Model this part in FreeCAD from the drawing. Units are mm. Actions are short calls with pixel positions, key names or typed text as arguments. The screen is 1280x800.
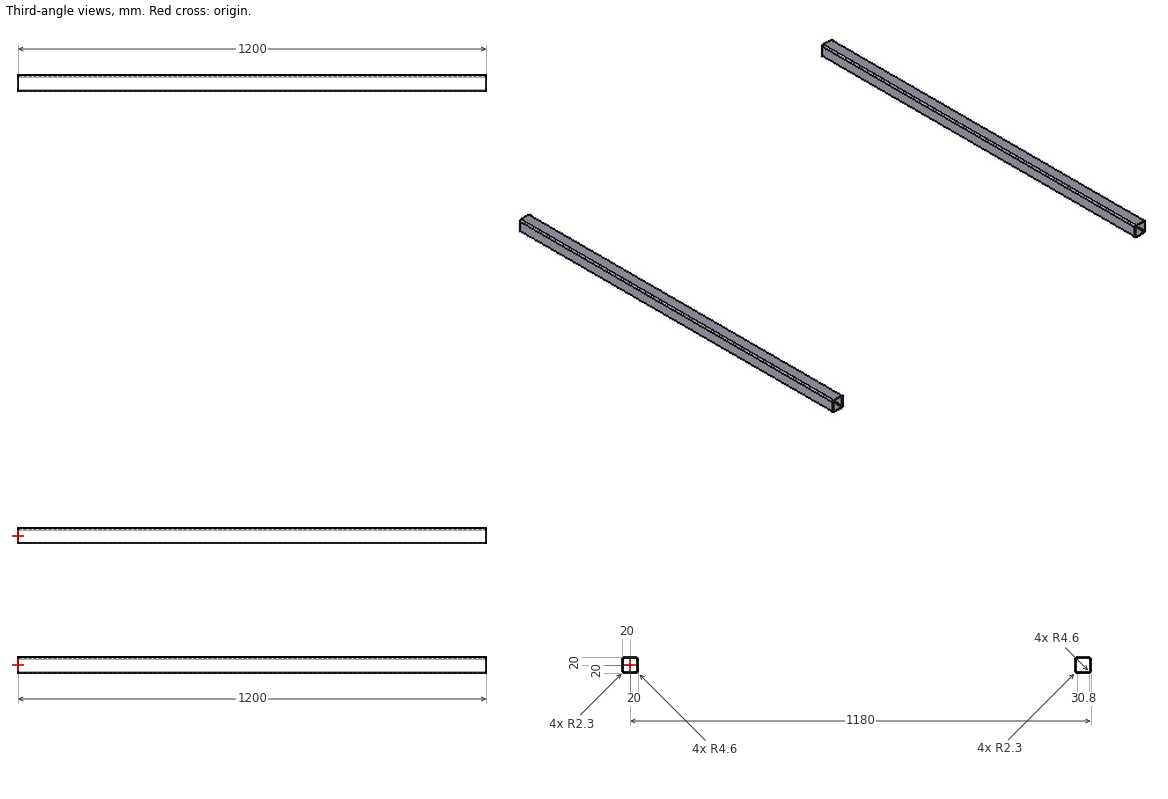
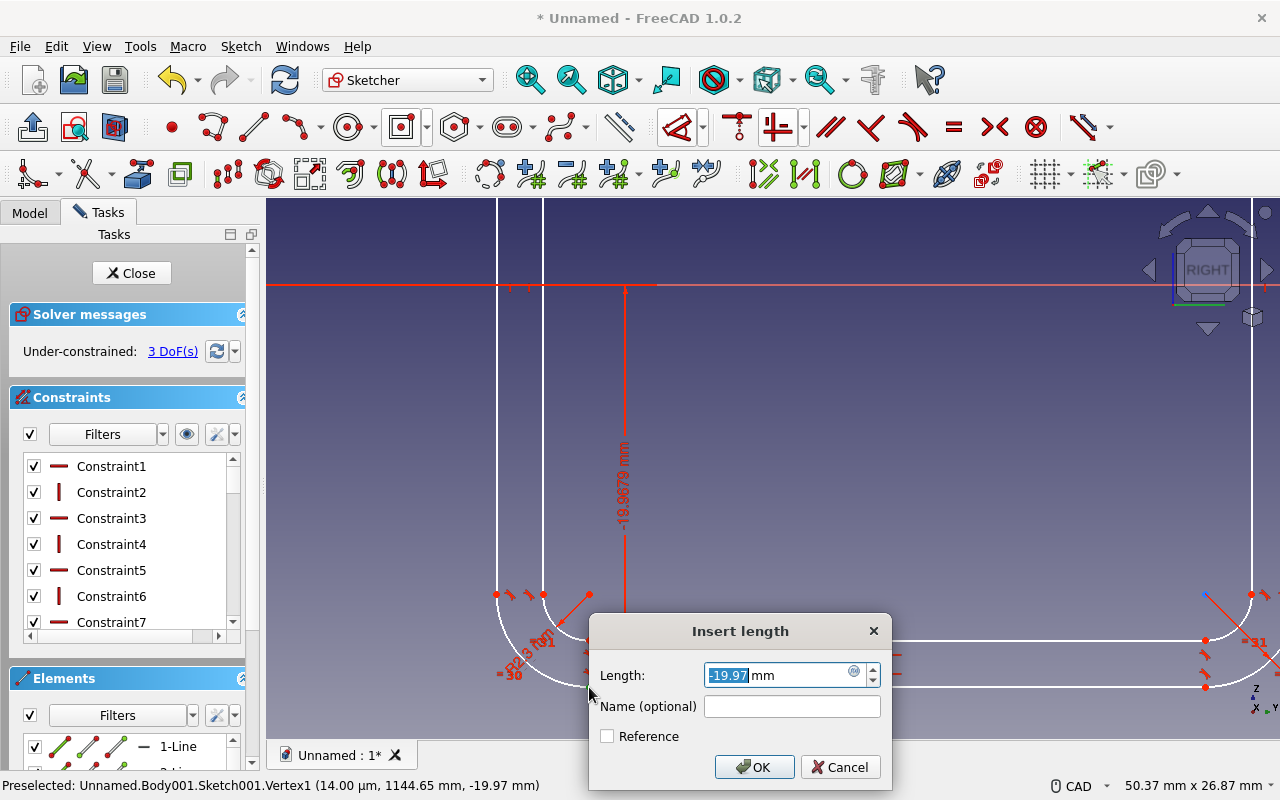
text(-20)
key(Return)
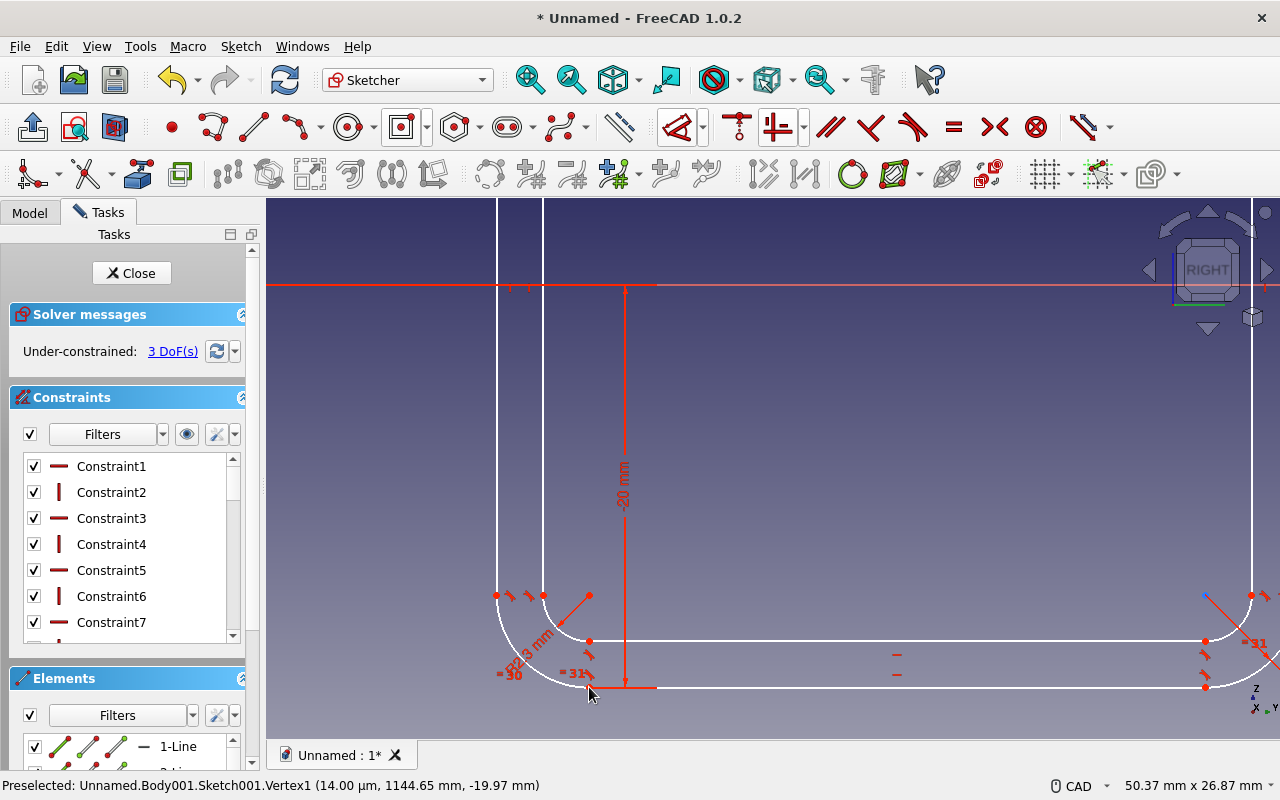
scroll(546, 618, down, 4)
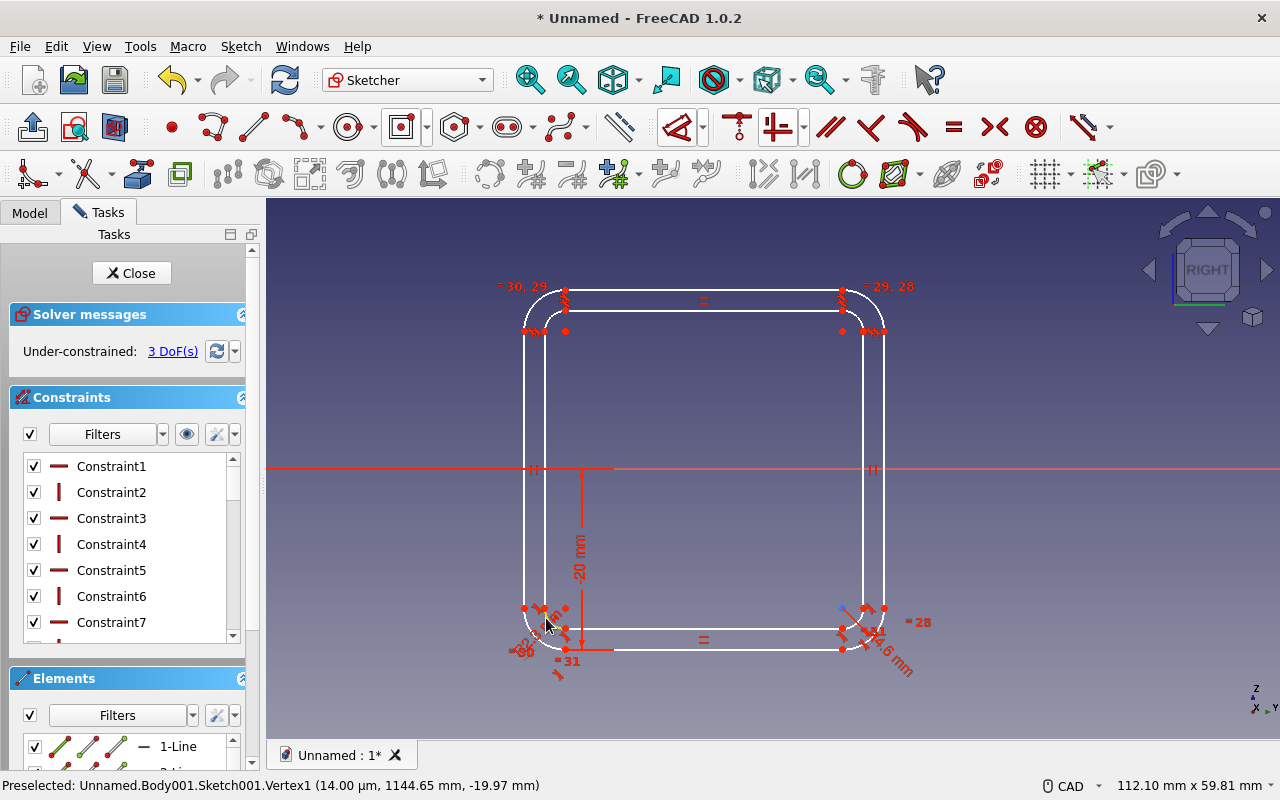
click(843, 290)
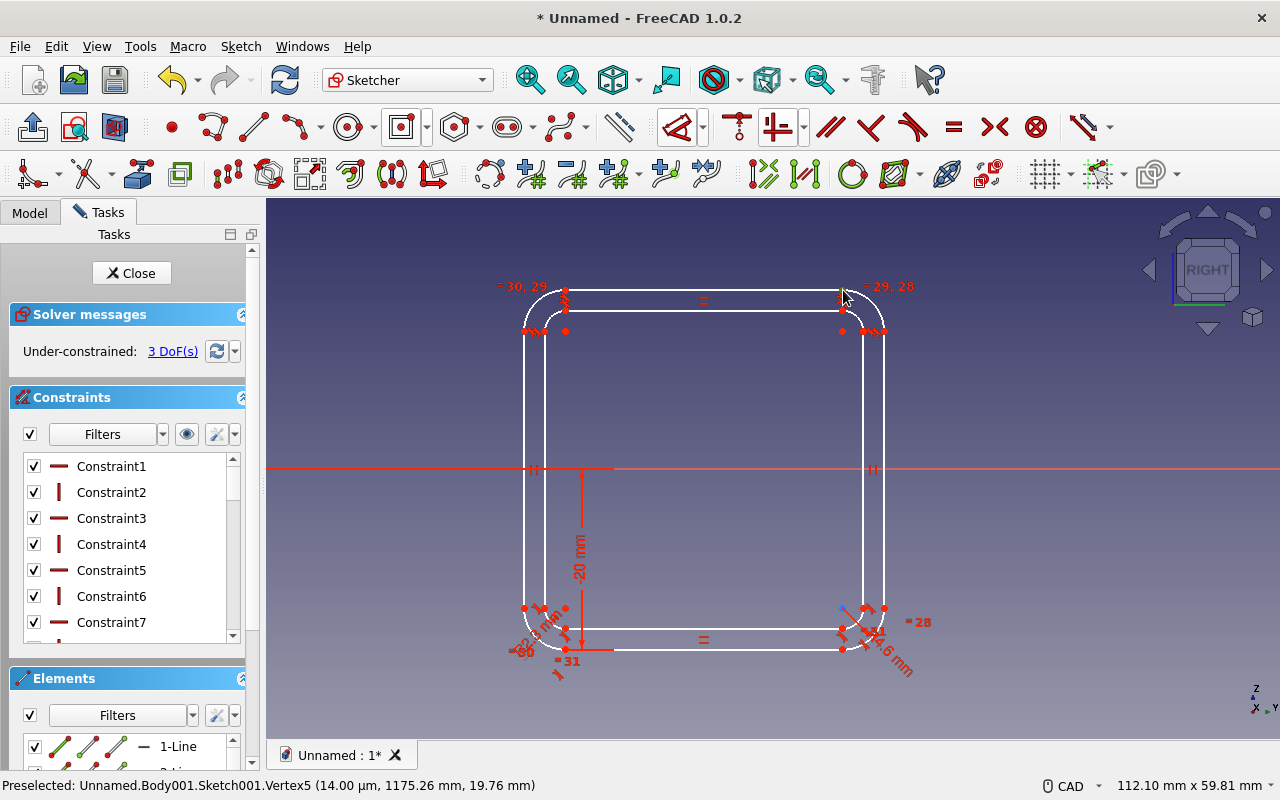
key(i)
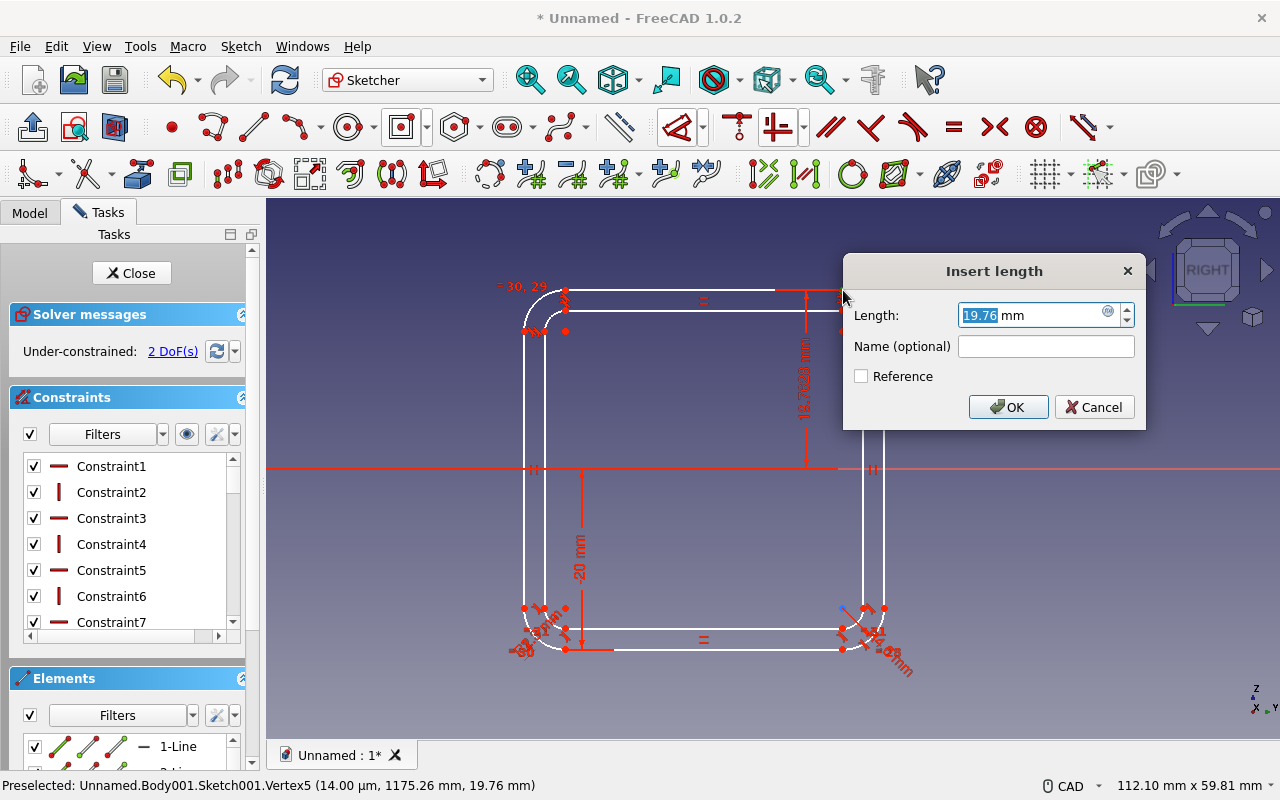
text(20)
key(Return)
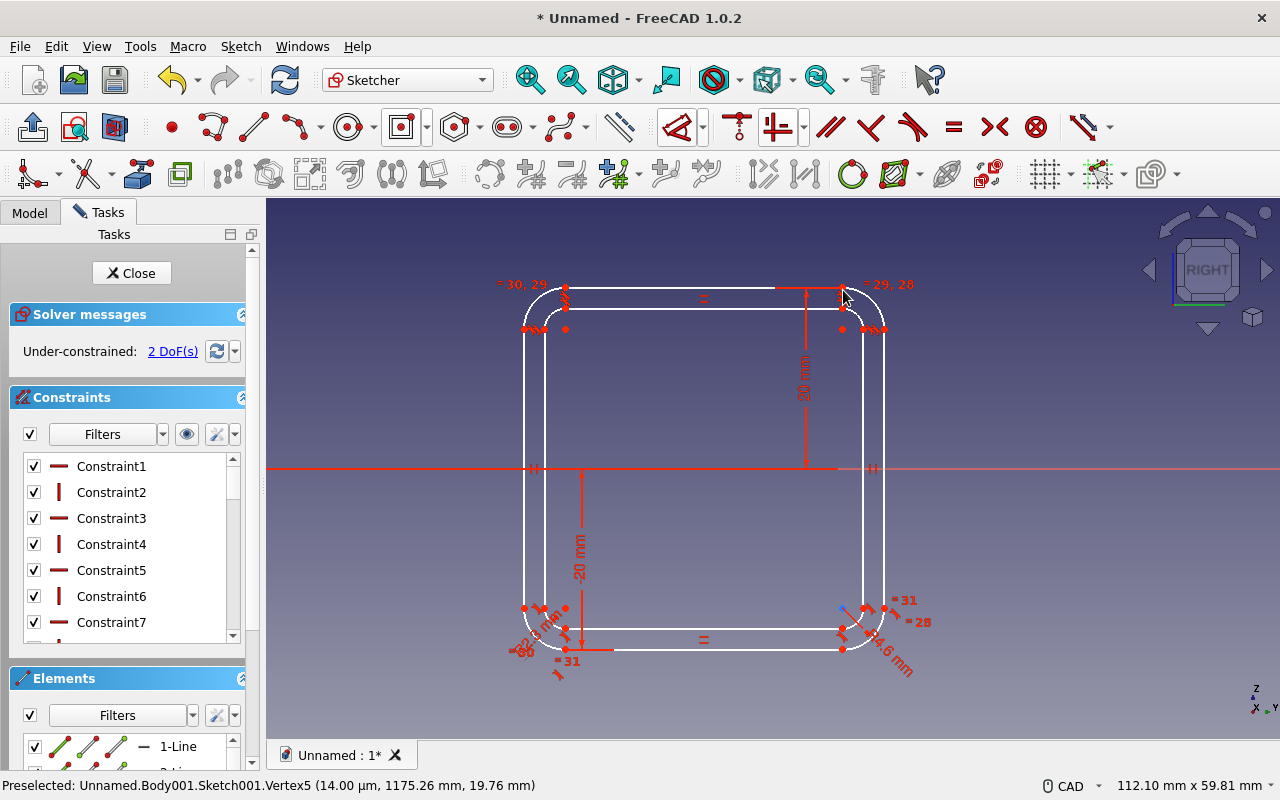
click(649, 650)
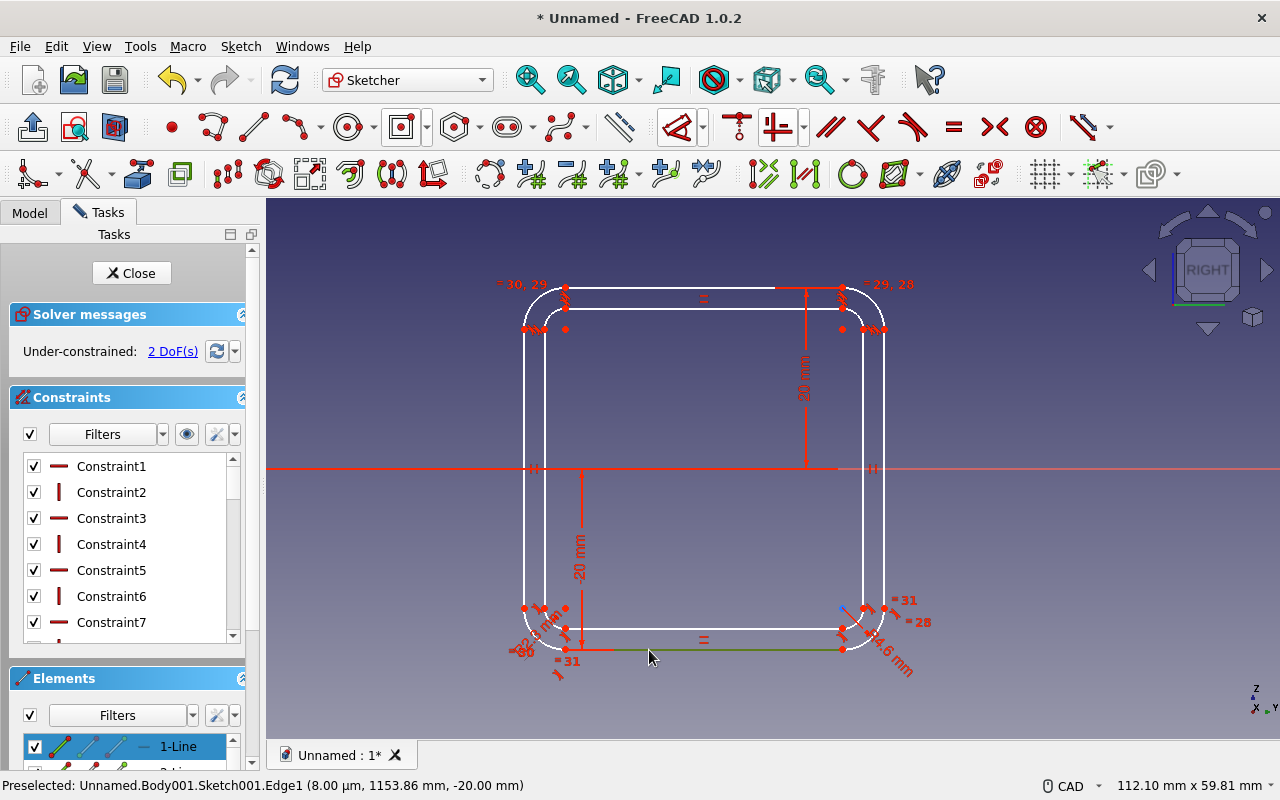
key(l)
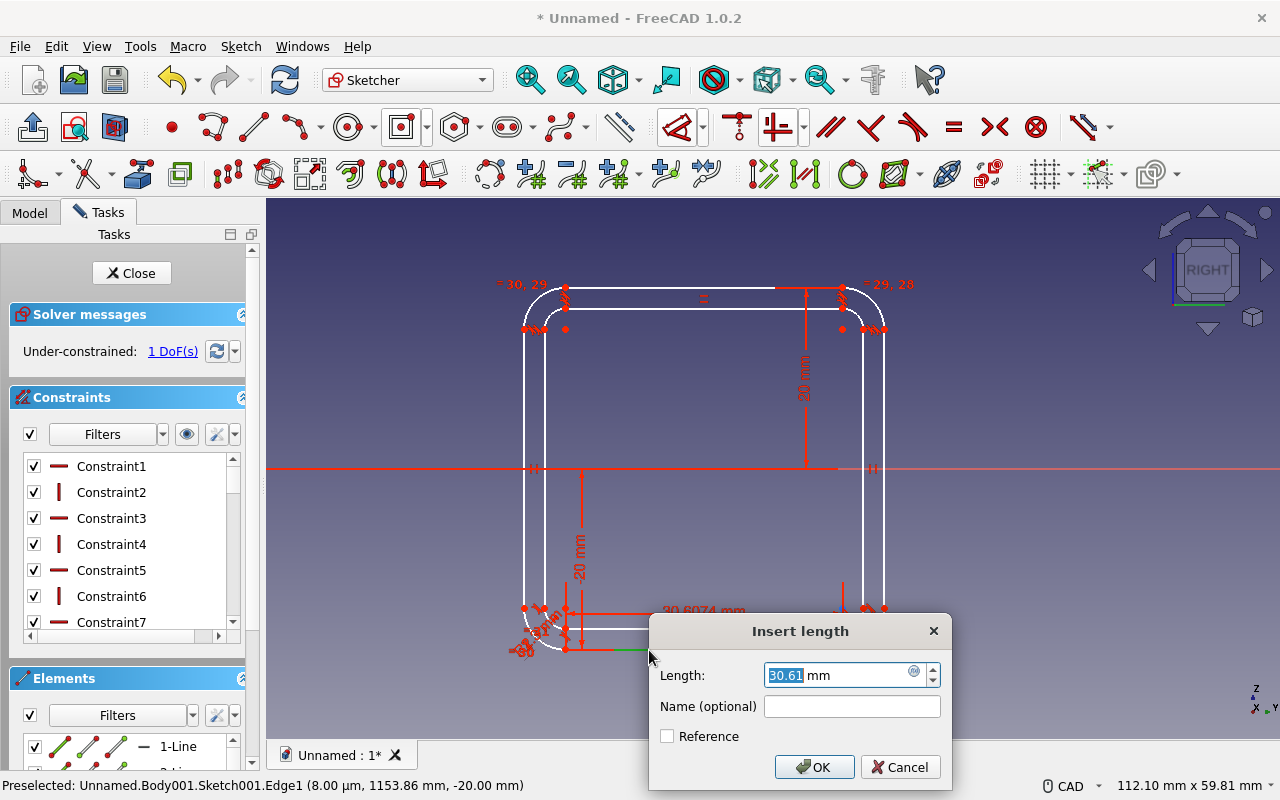
text(30.8)
key(Return)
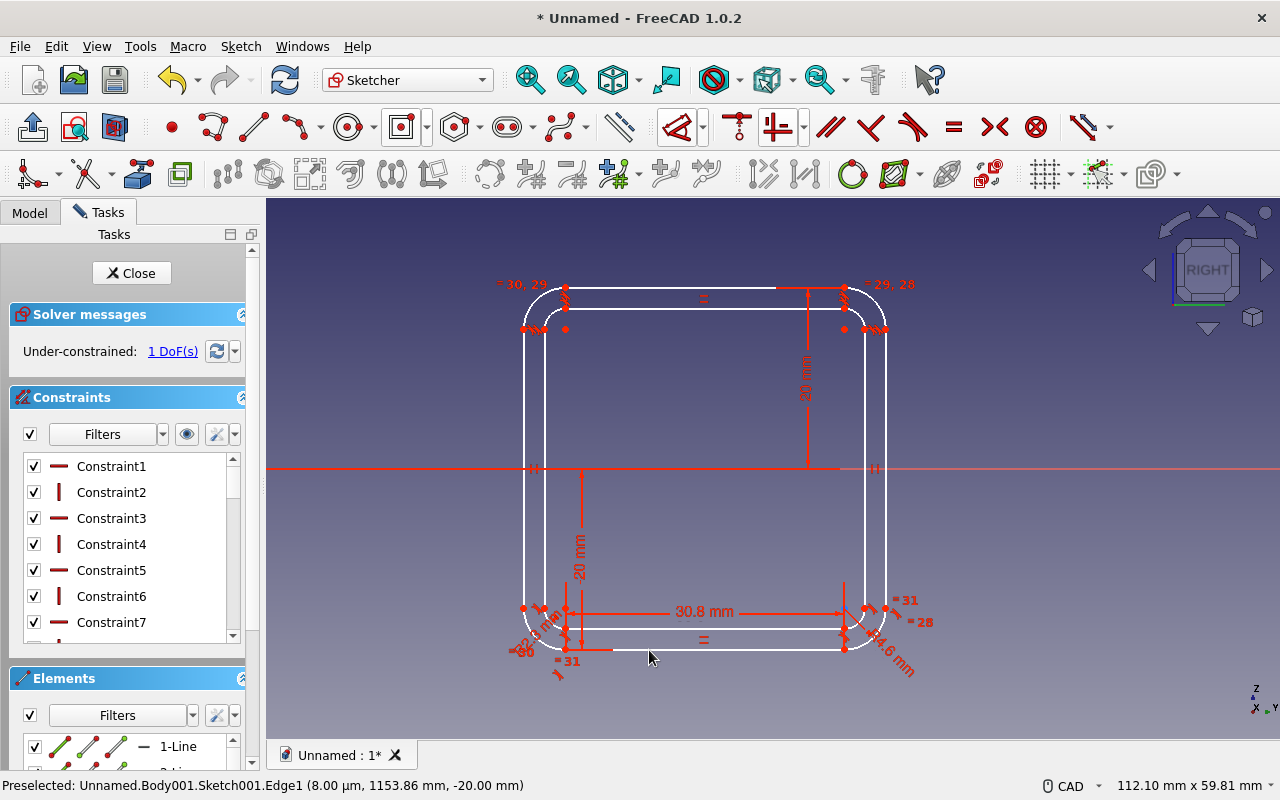
click(886, 608)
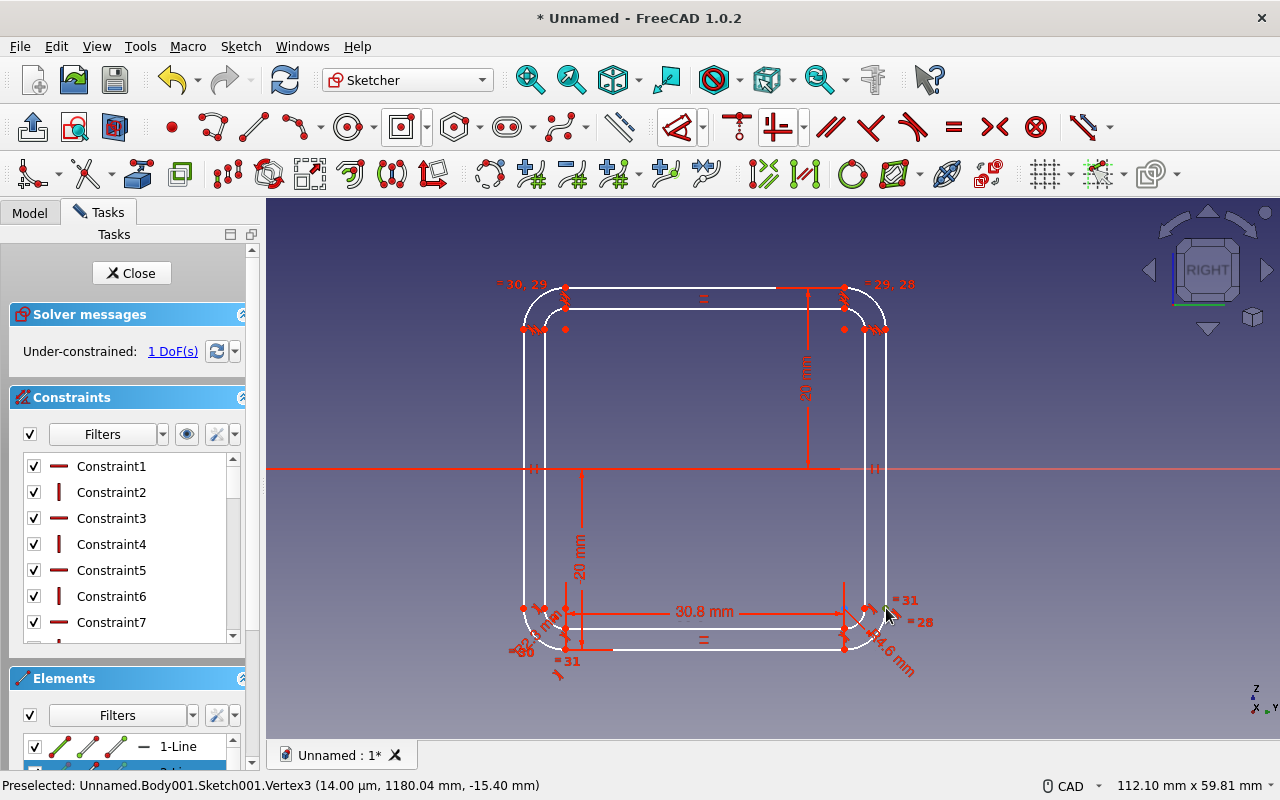
key(l)